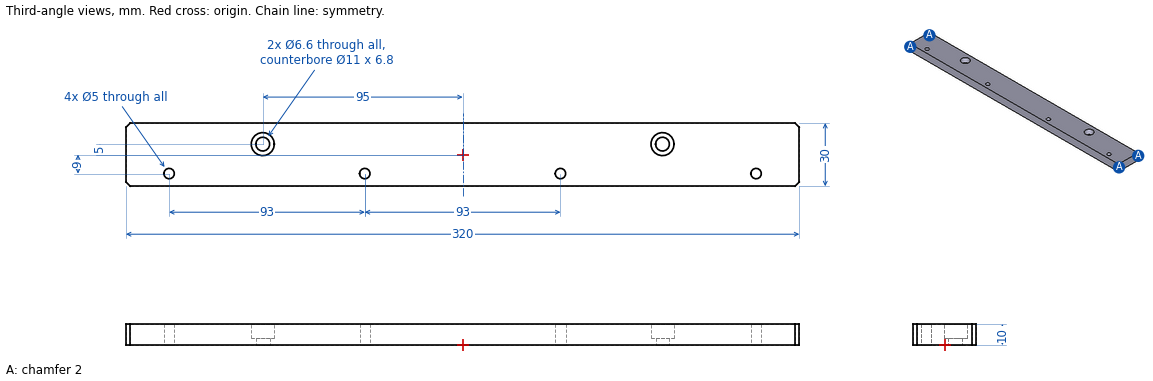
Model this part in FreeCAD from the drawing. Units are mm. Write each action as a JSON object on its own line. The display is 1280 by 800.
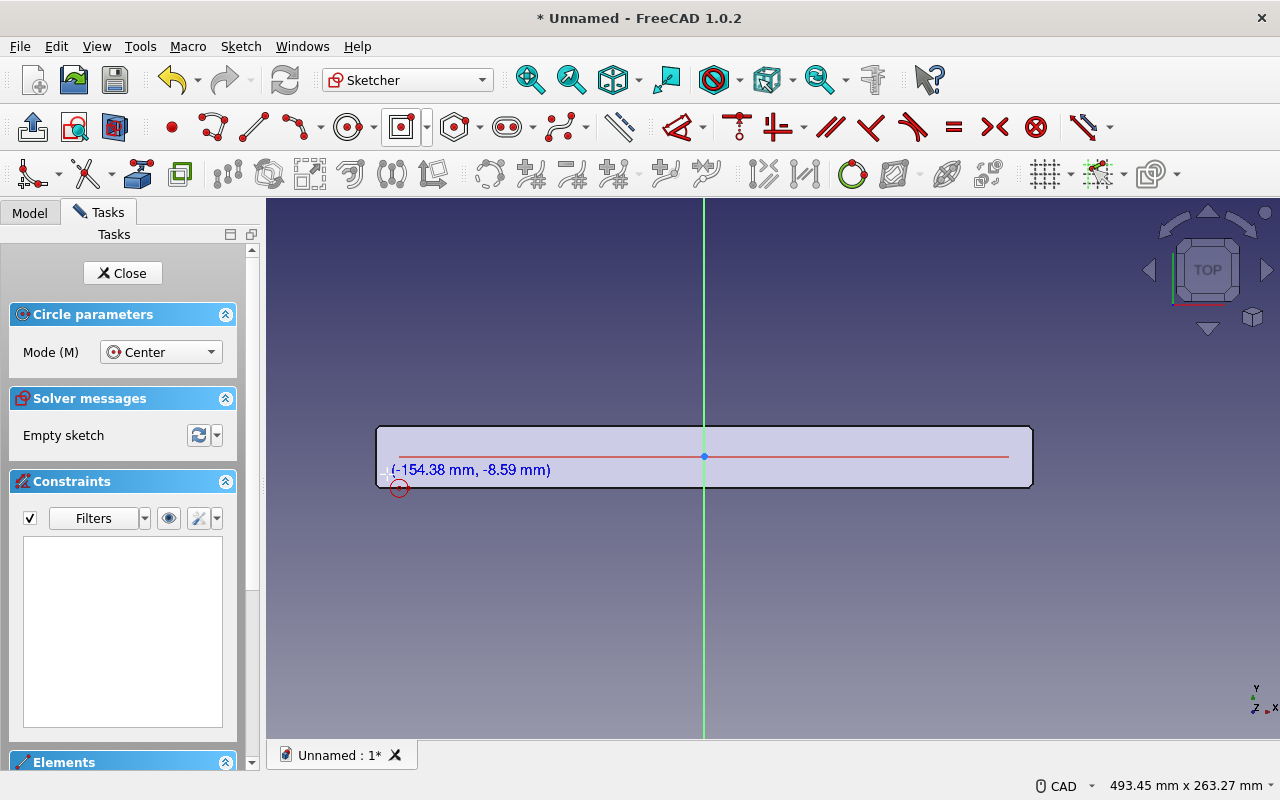
{"action": "left_click", "coordinate": [418, 475]}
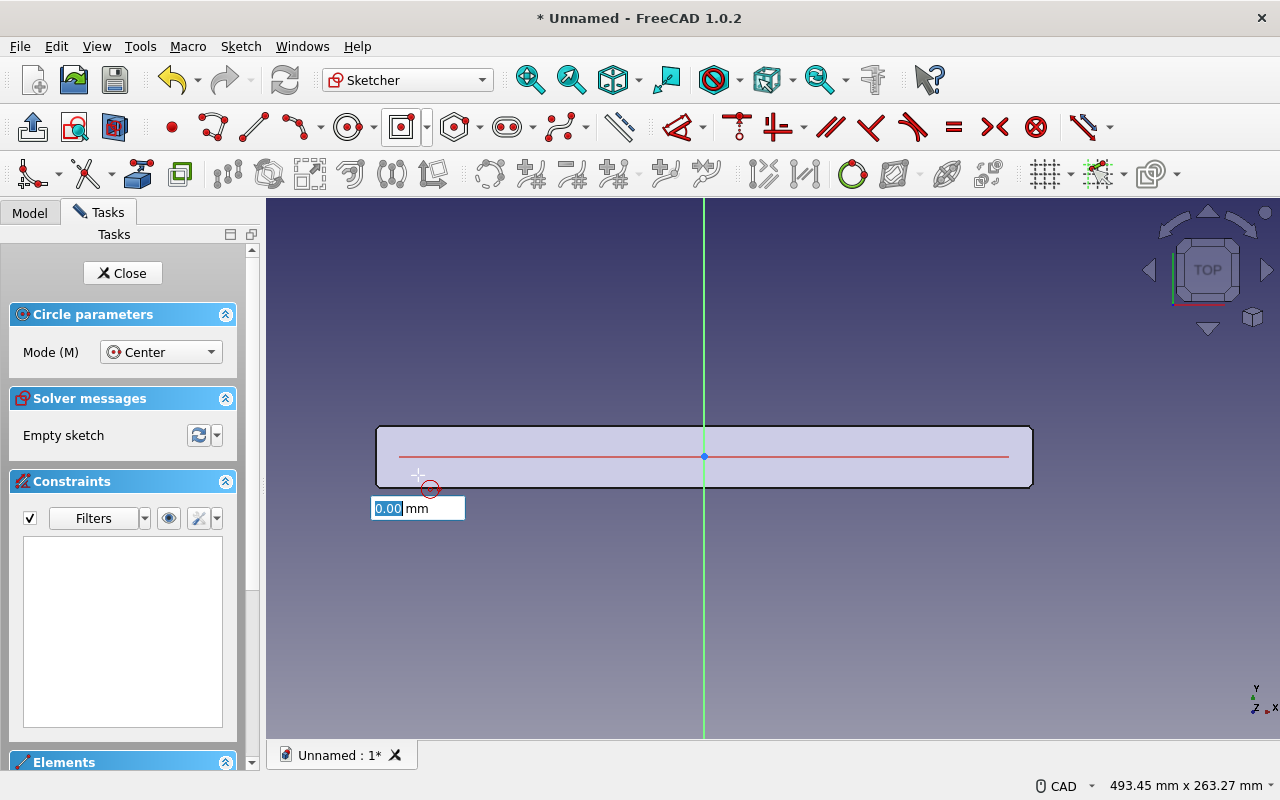
{"action": "scroll", "coordinate": [421, 472], "scroll_direction": "up", "scroll_amount": 6}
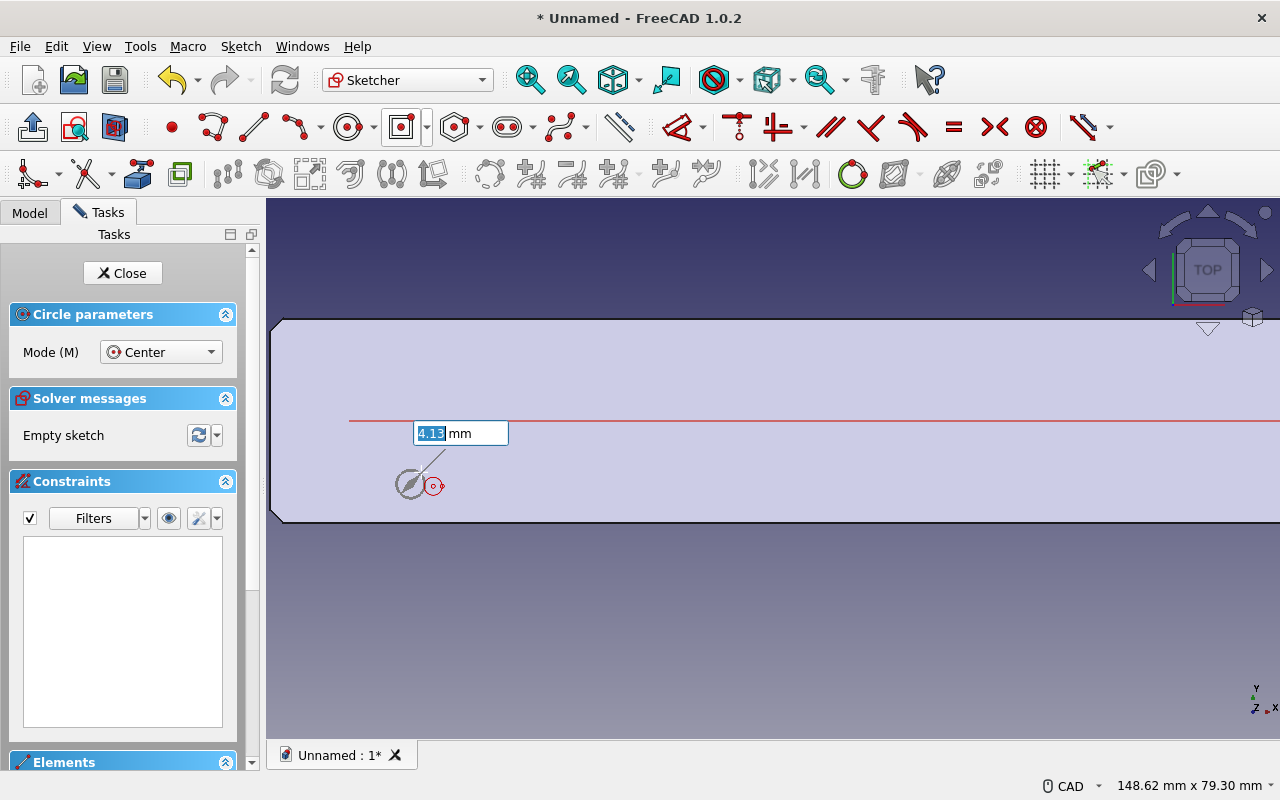
{"action": "left_click", "coordinate": [422, 470]}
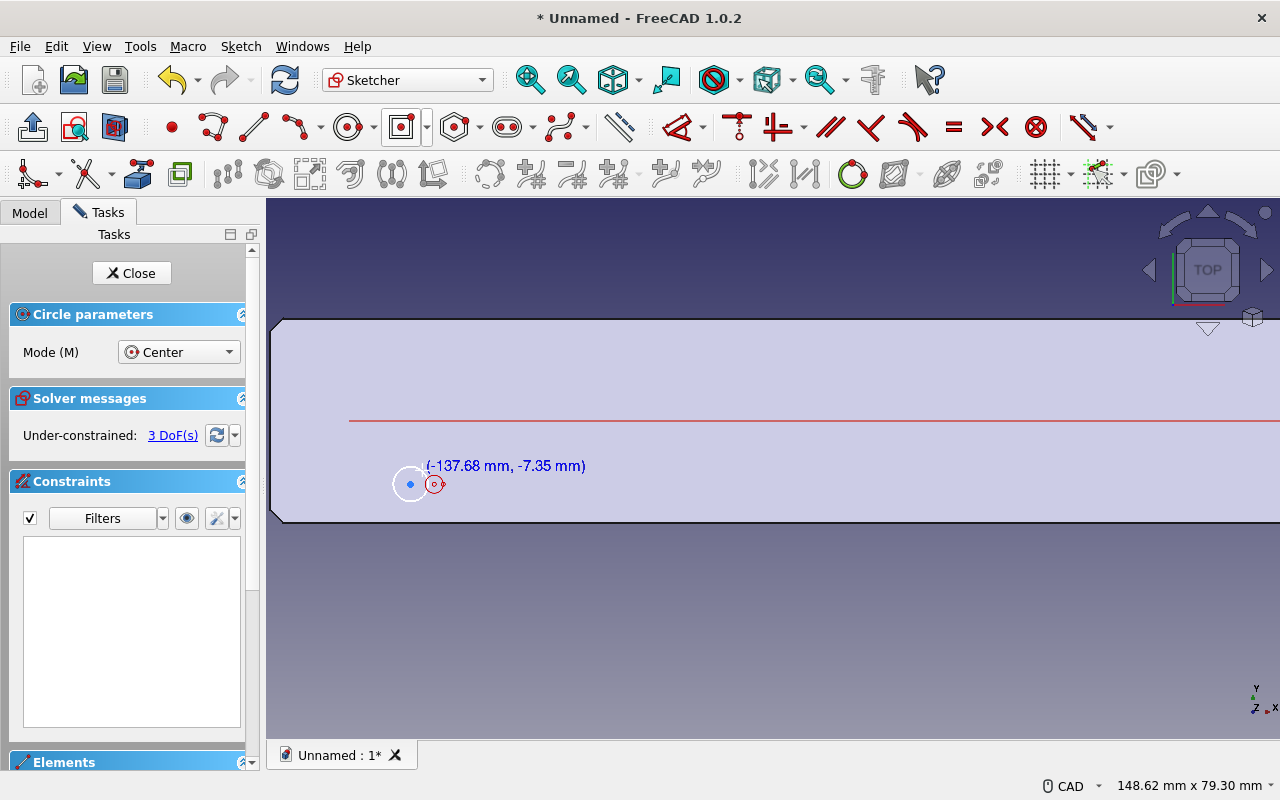
{"action": "scroll", "coordinate": [1044, 482], "scroll_direction": "up", "scroll_amount": 2}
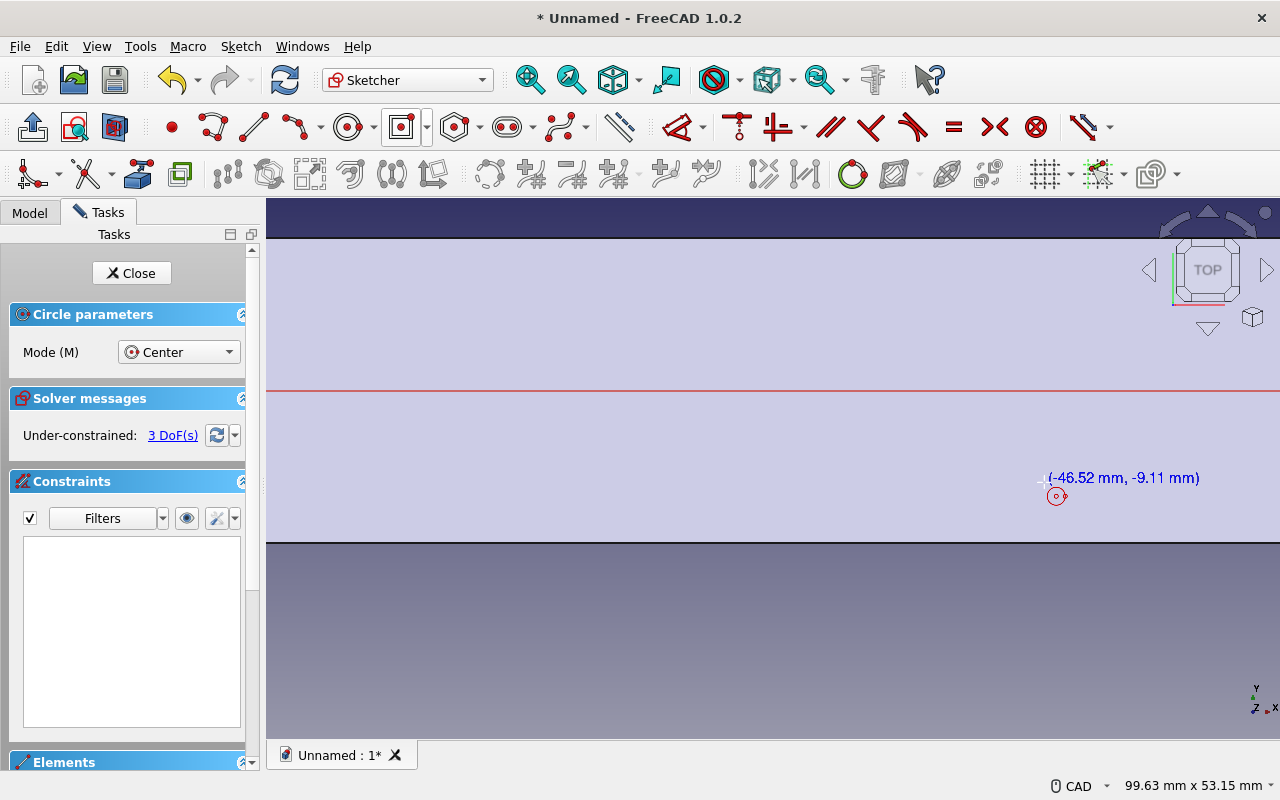
{"action": "scroll", "coordinate": [499, 473], "scroll_direction": "down", "scroll_amount": 8}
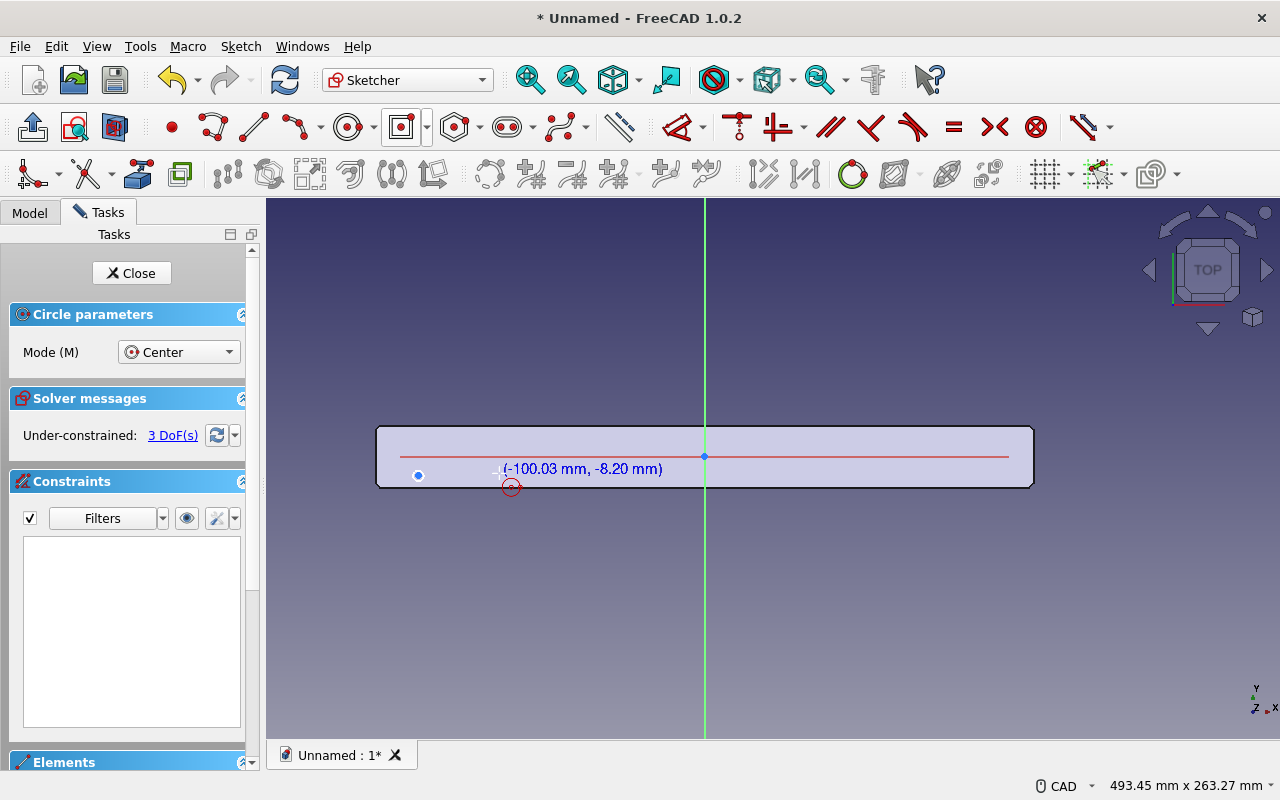
{"action": "left_click", "coordinate": [609, 475]}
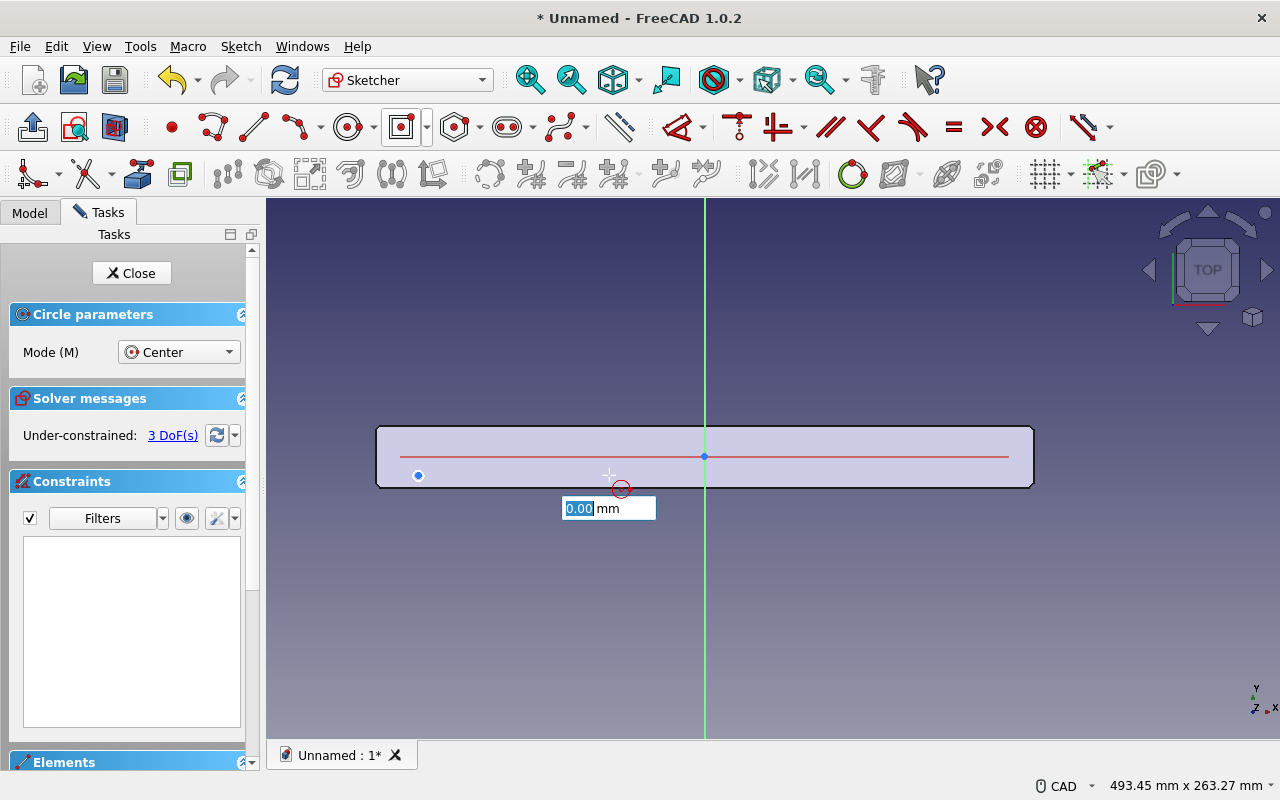
{"action": "scroll", "coordinate": [613, 472], "scroll_direction": "up", "scroll_amount": 6}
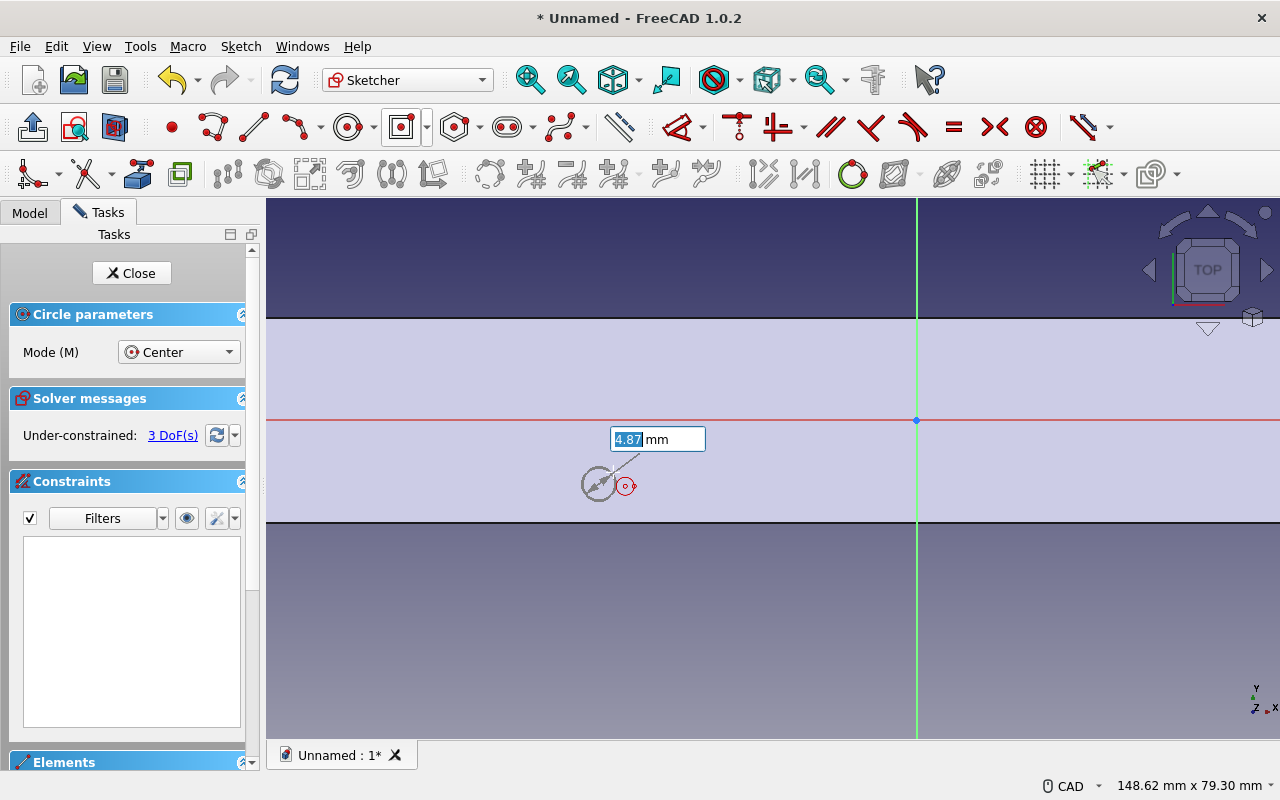
{"action": "left_click", "coordinate": [612, 470]}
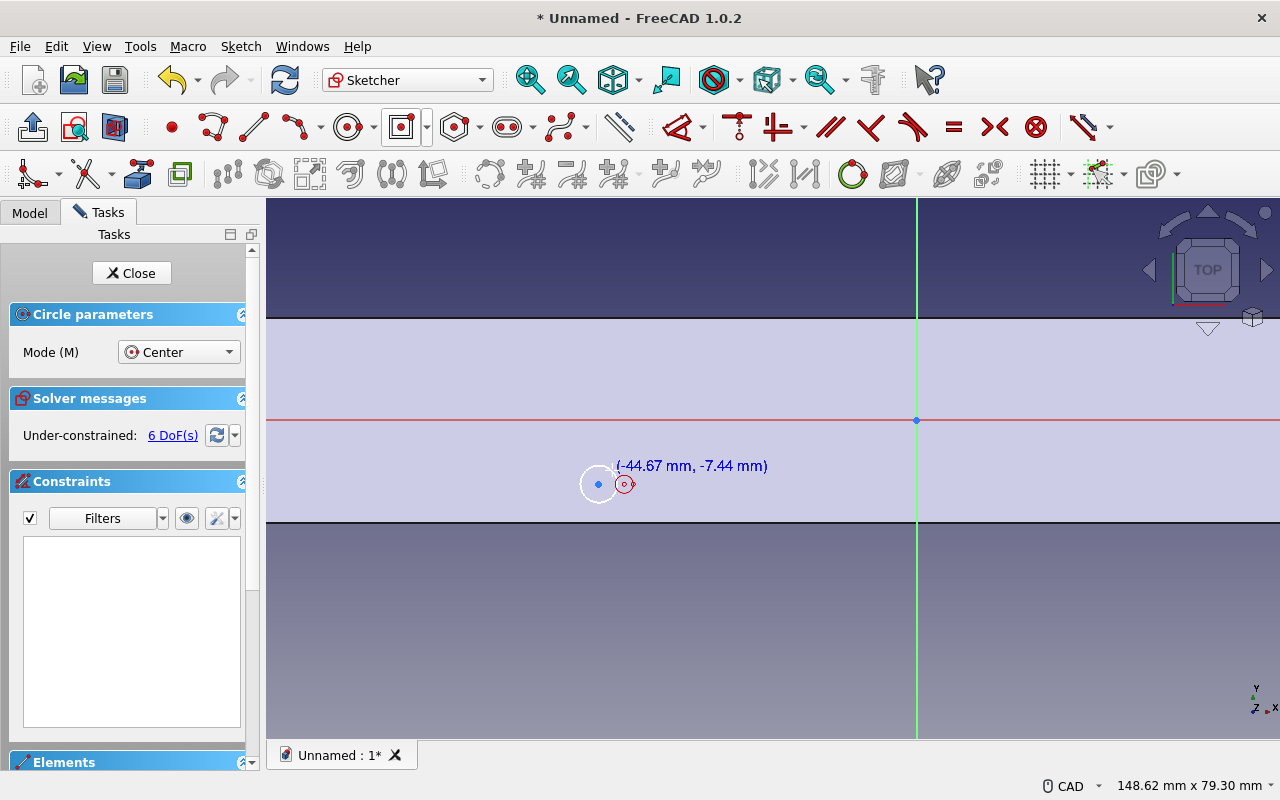
{"action": "scroll", "coordinate": [613, 472], "scroll_direction": "down", "scroll_amount": 6}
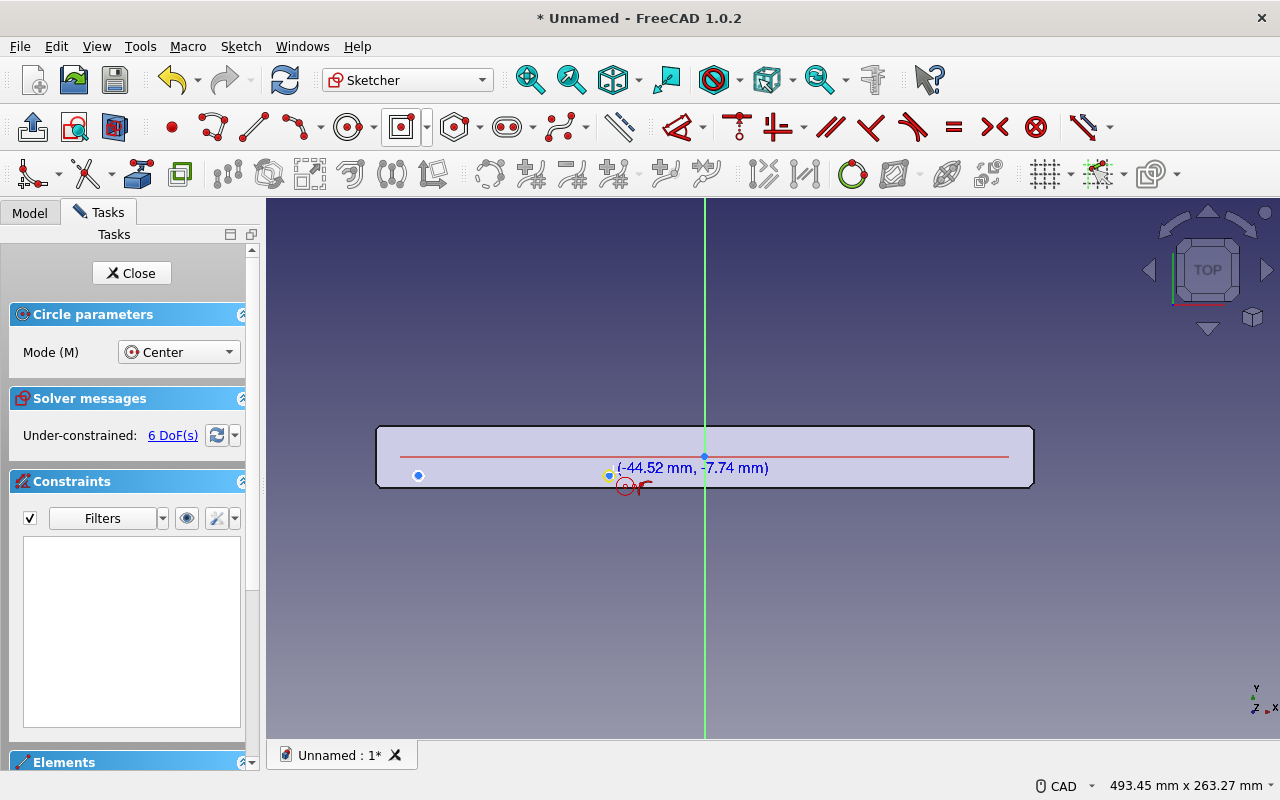
{"action": "scroll", "coordinate": [800, 475], "scroll_direction": "up", "scroll_amount": 8}